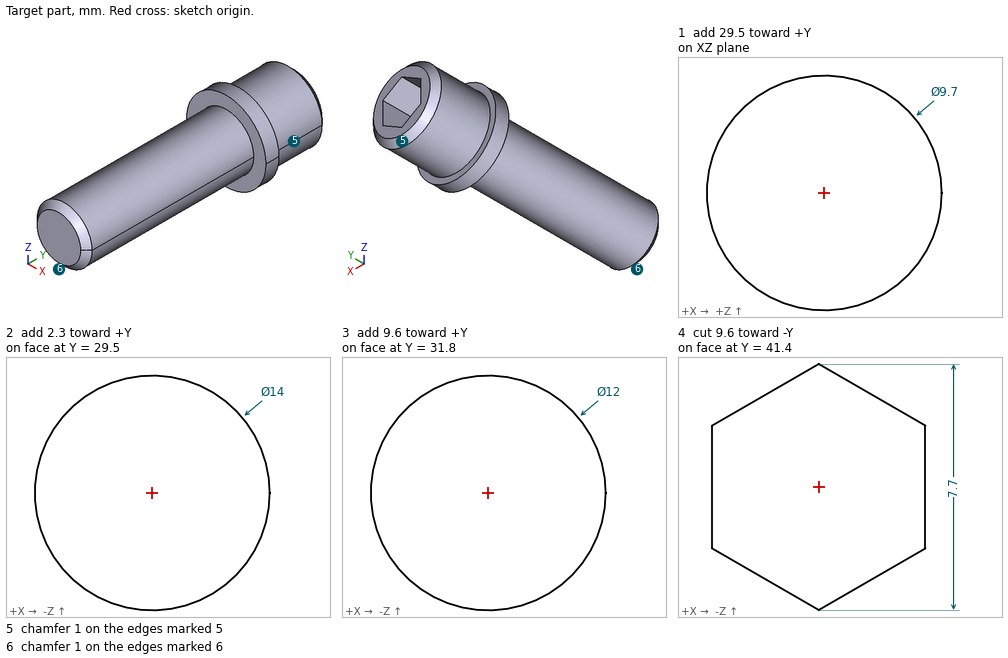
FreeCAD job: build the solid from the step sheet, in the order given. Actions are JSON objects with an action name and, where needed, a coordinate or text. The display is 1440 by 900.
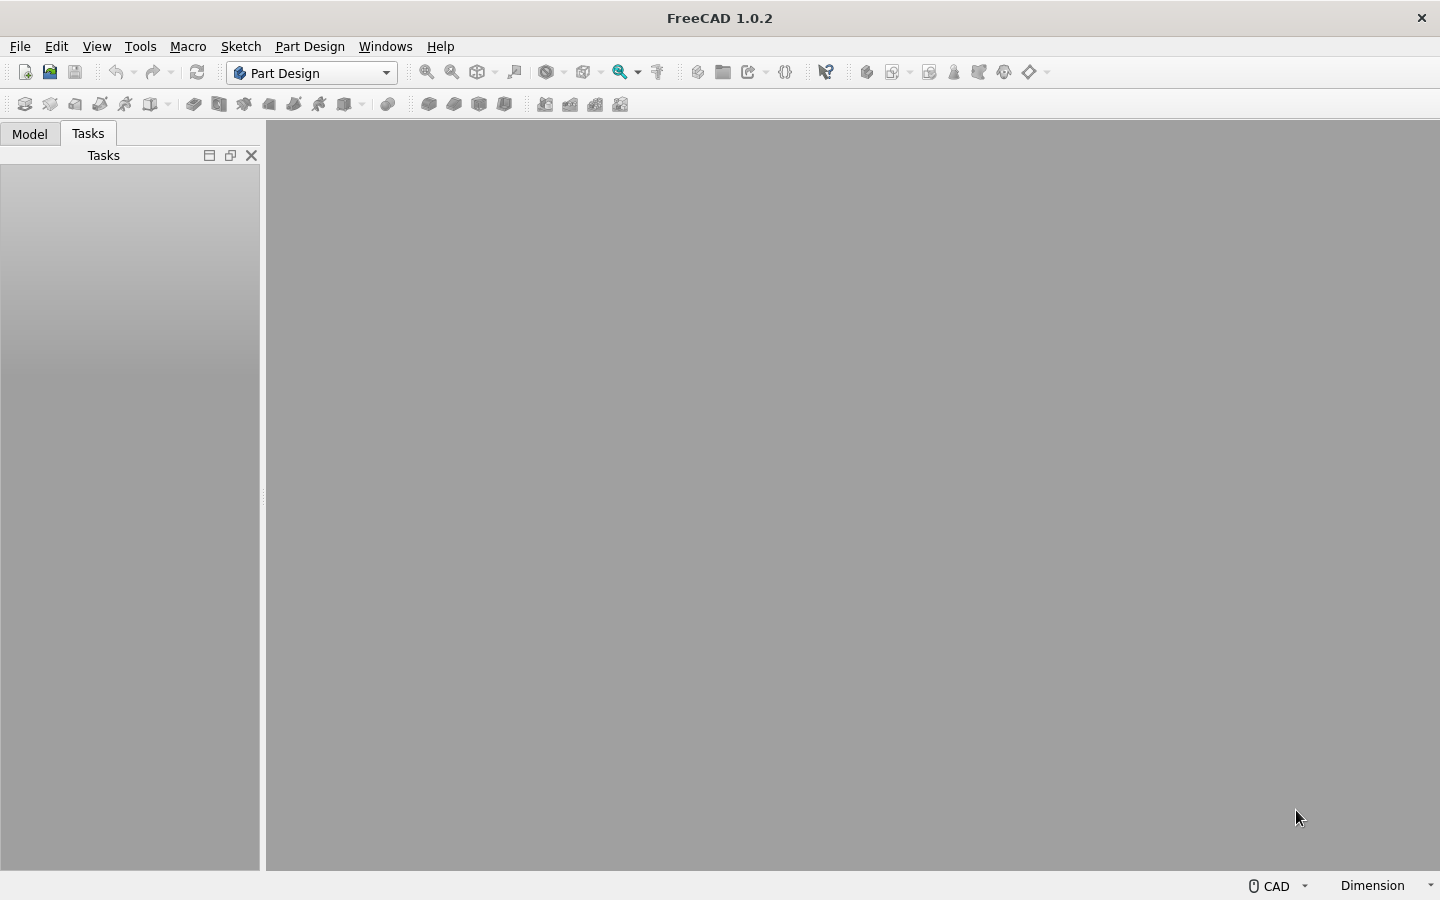
{"action": "left_click", "coordinate": [25, 72]}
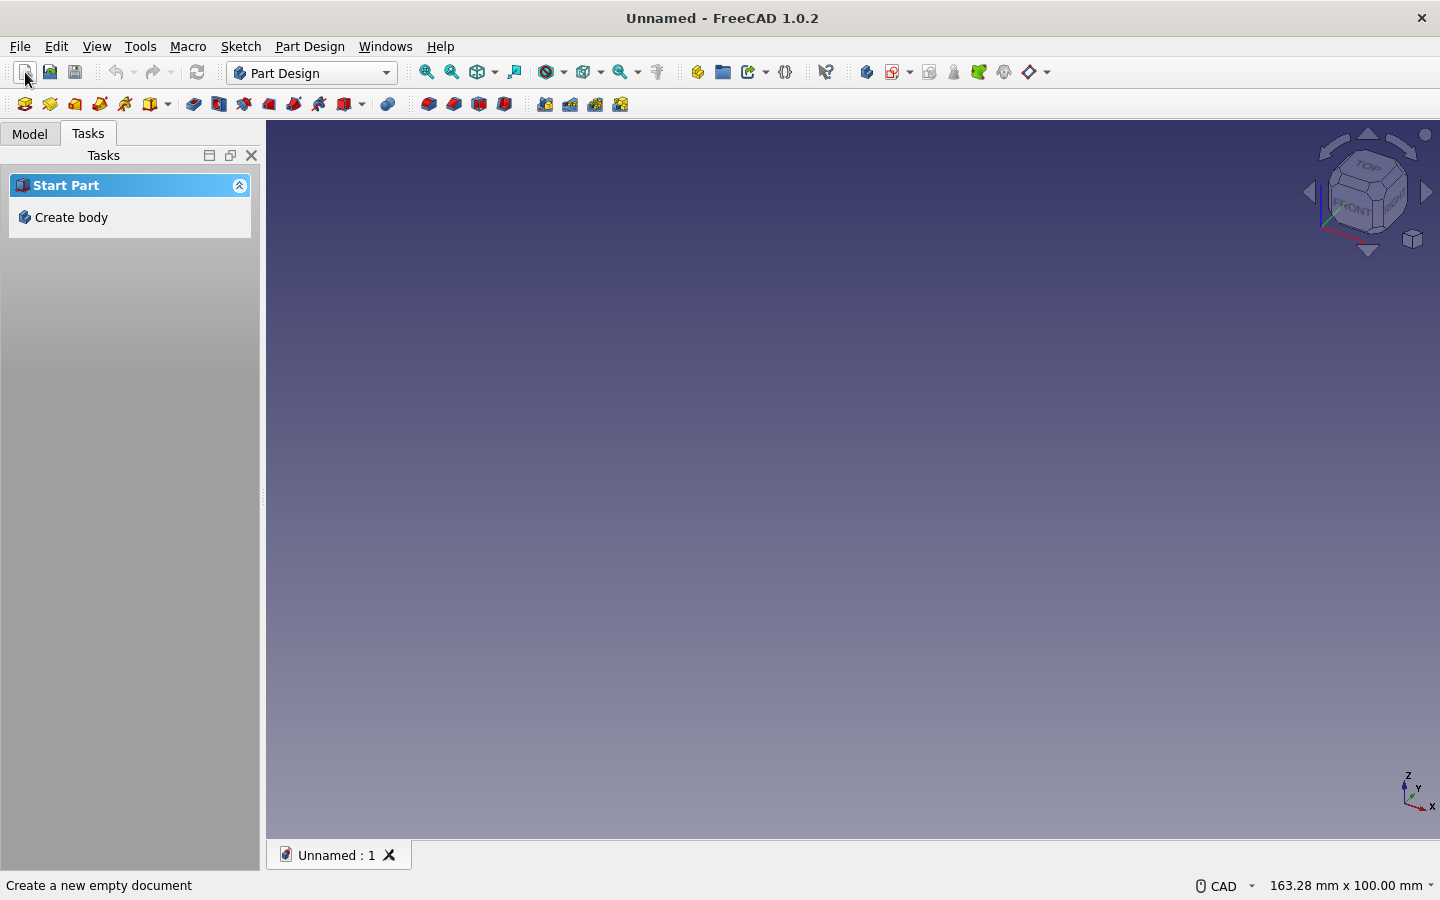
{"action": "left_click", "coordinate": [892, 72]}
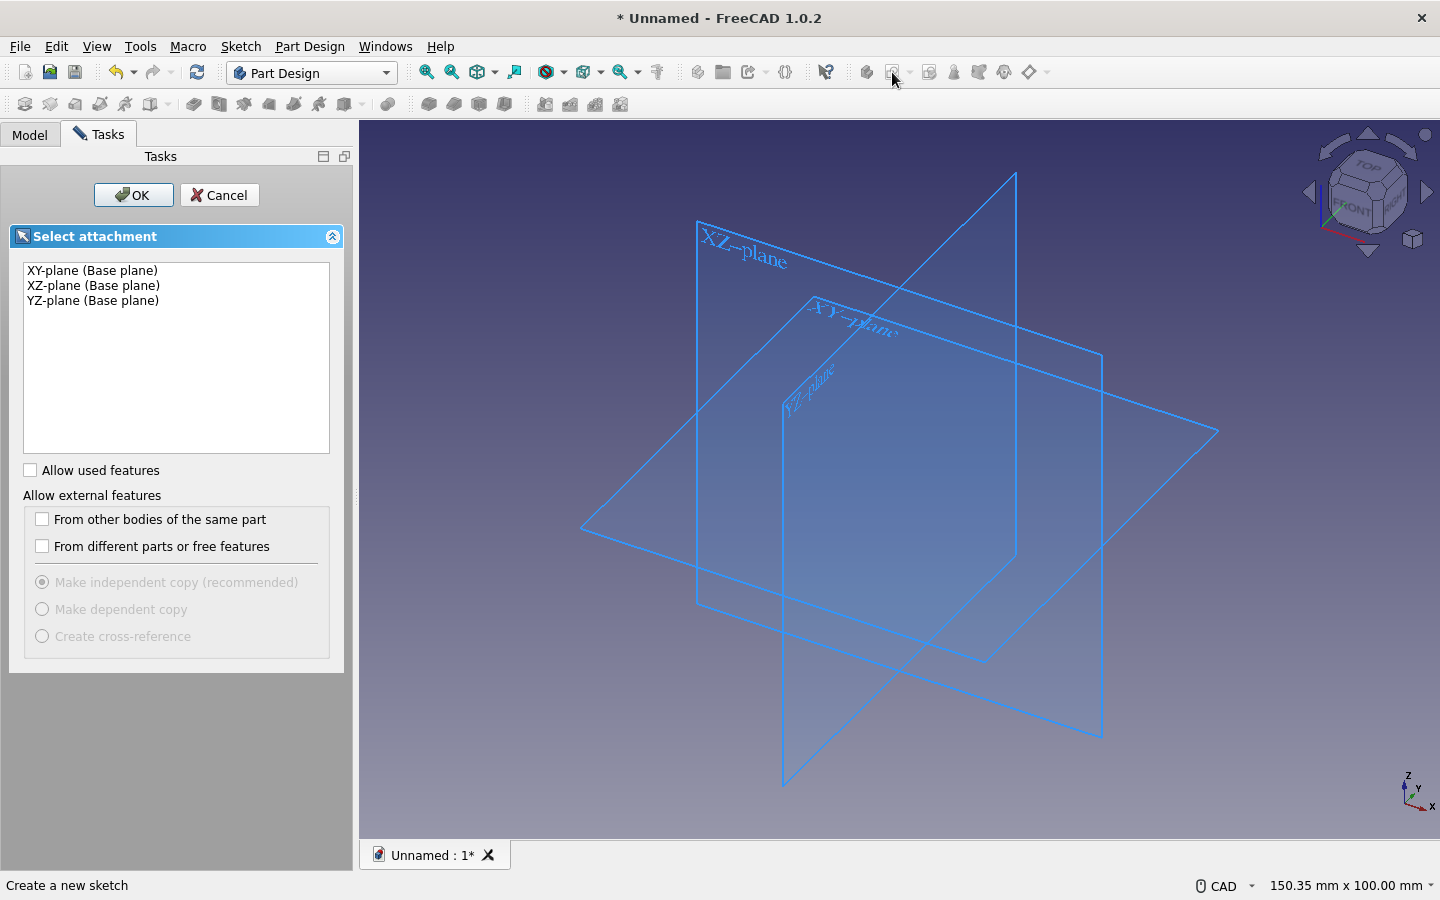
{"action": "left_click", "coordinate": [84, 286]}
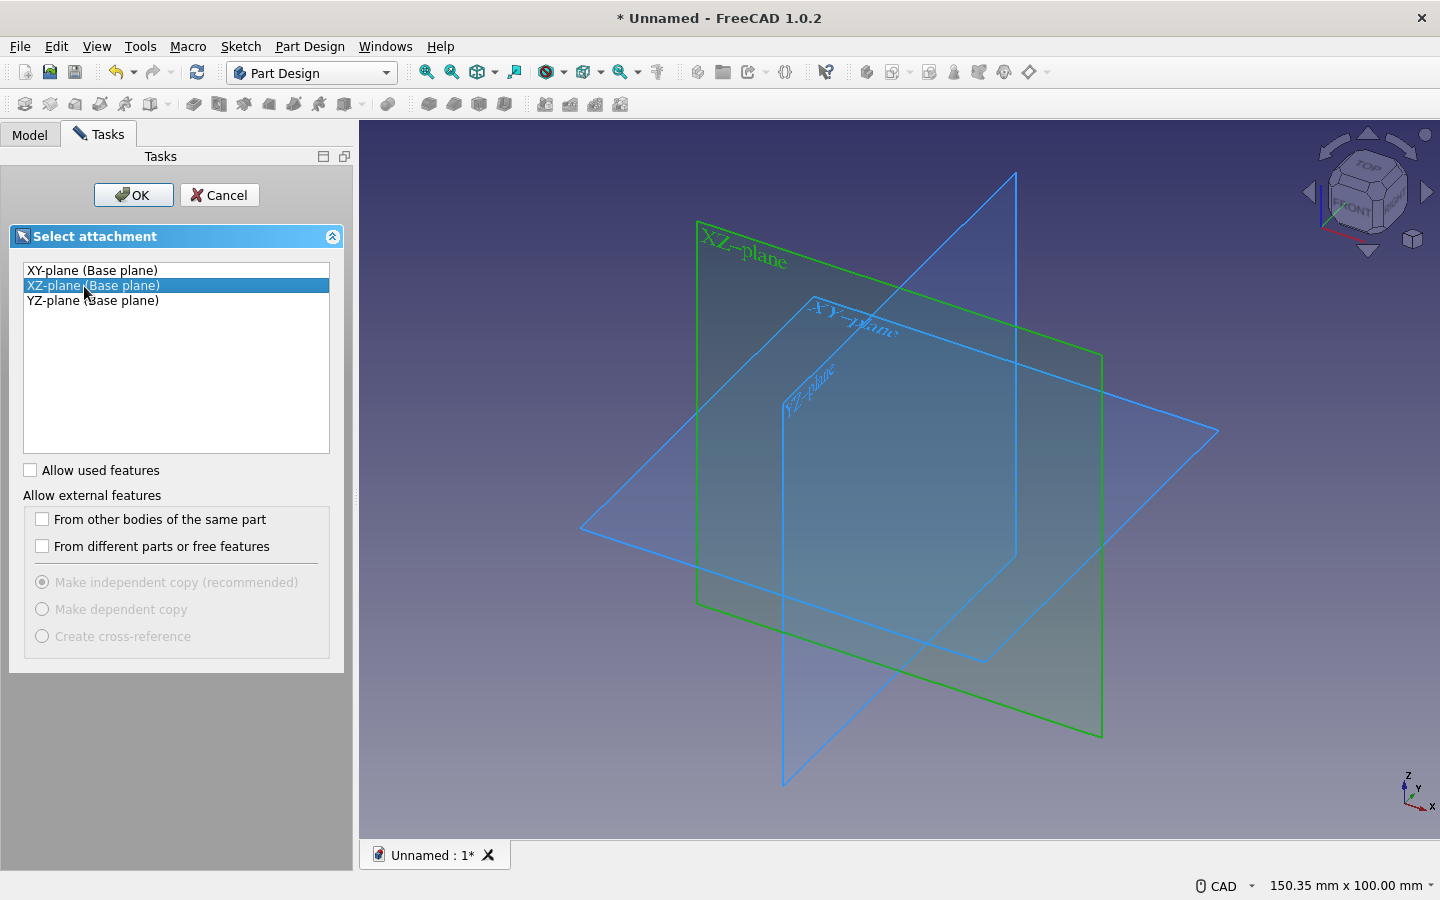
{"action": "left_click", "coordinate": [134, 195]}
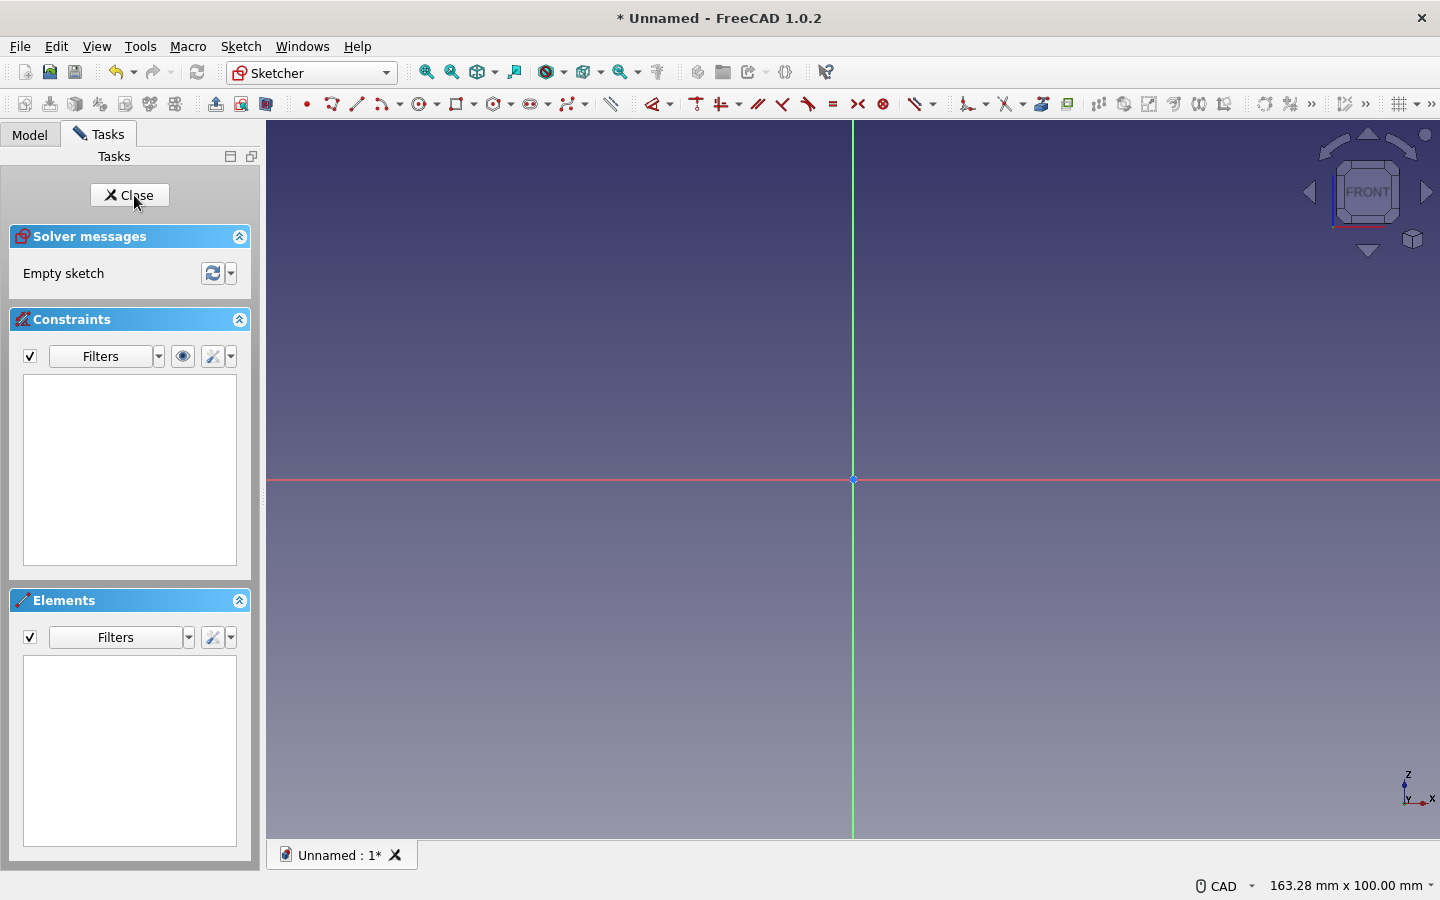
{"action": "scroll", "coordinate": [864, 480], "scroll_direction": "up", "scroll_amount": 10}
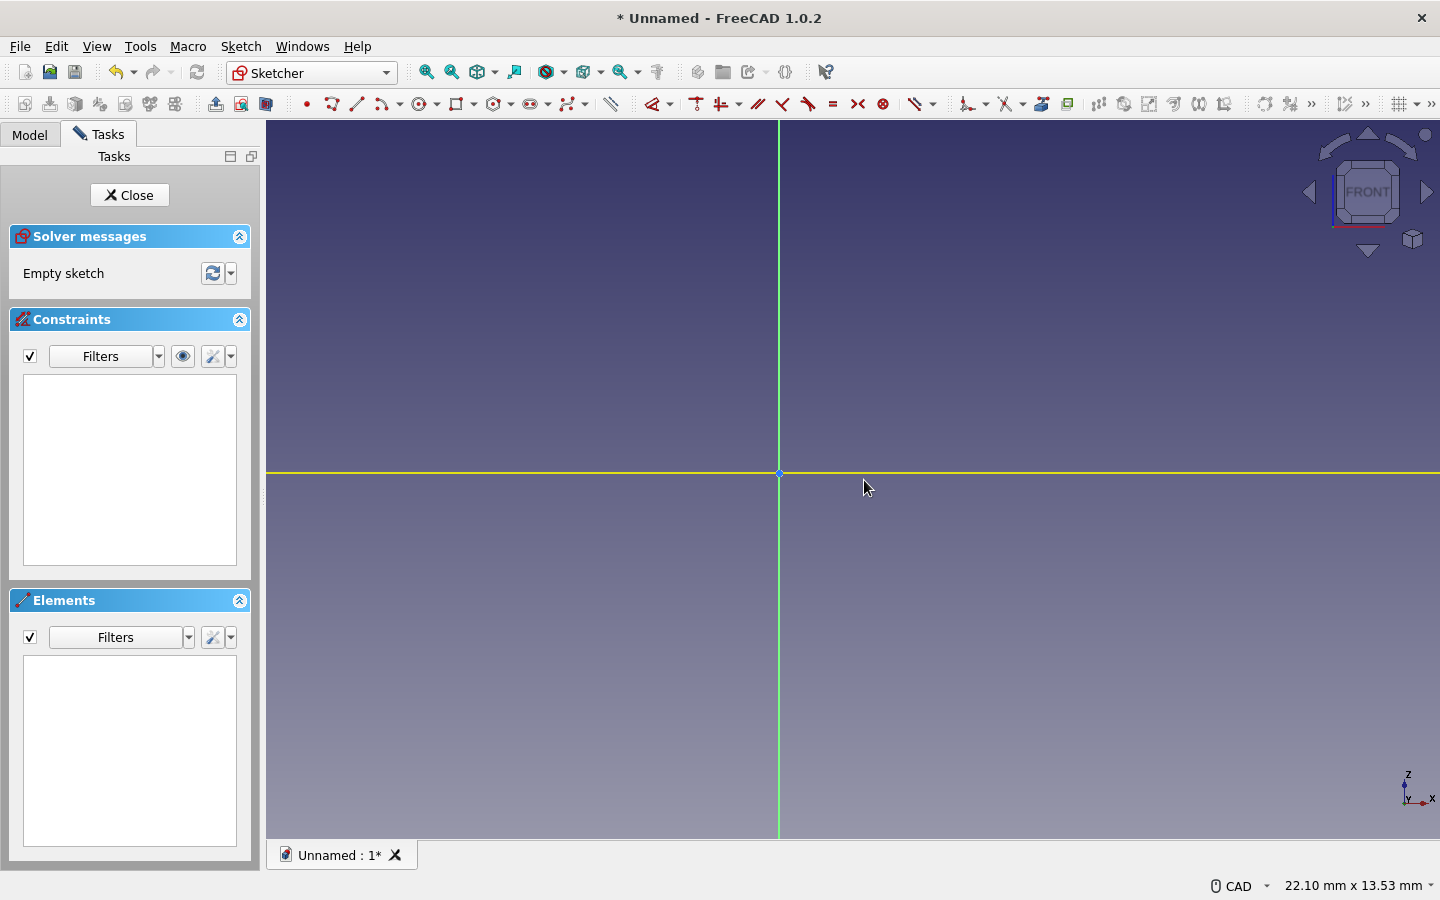
{"action": "left_click", "coordinate": [418, 104]}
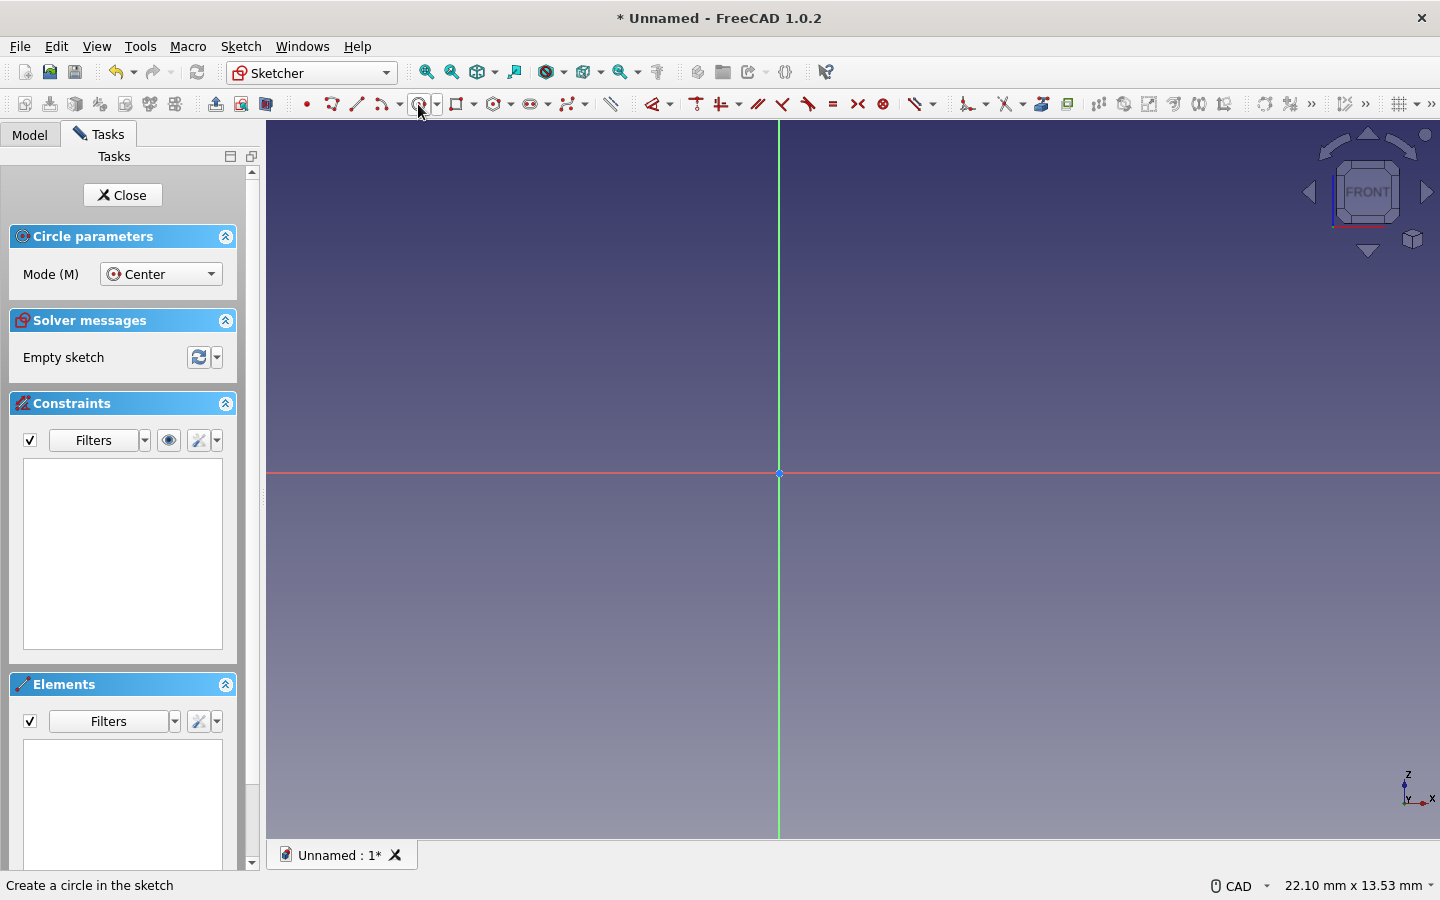
{"action": "left_click", "coordinate": [779, 473]}
{"action": "mouse_move", "coordinate": [962, 291]}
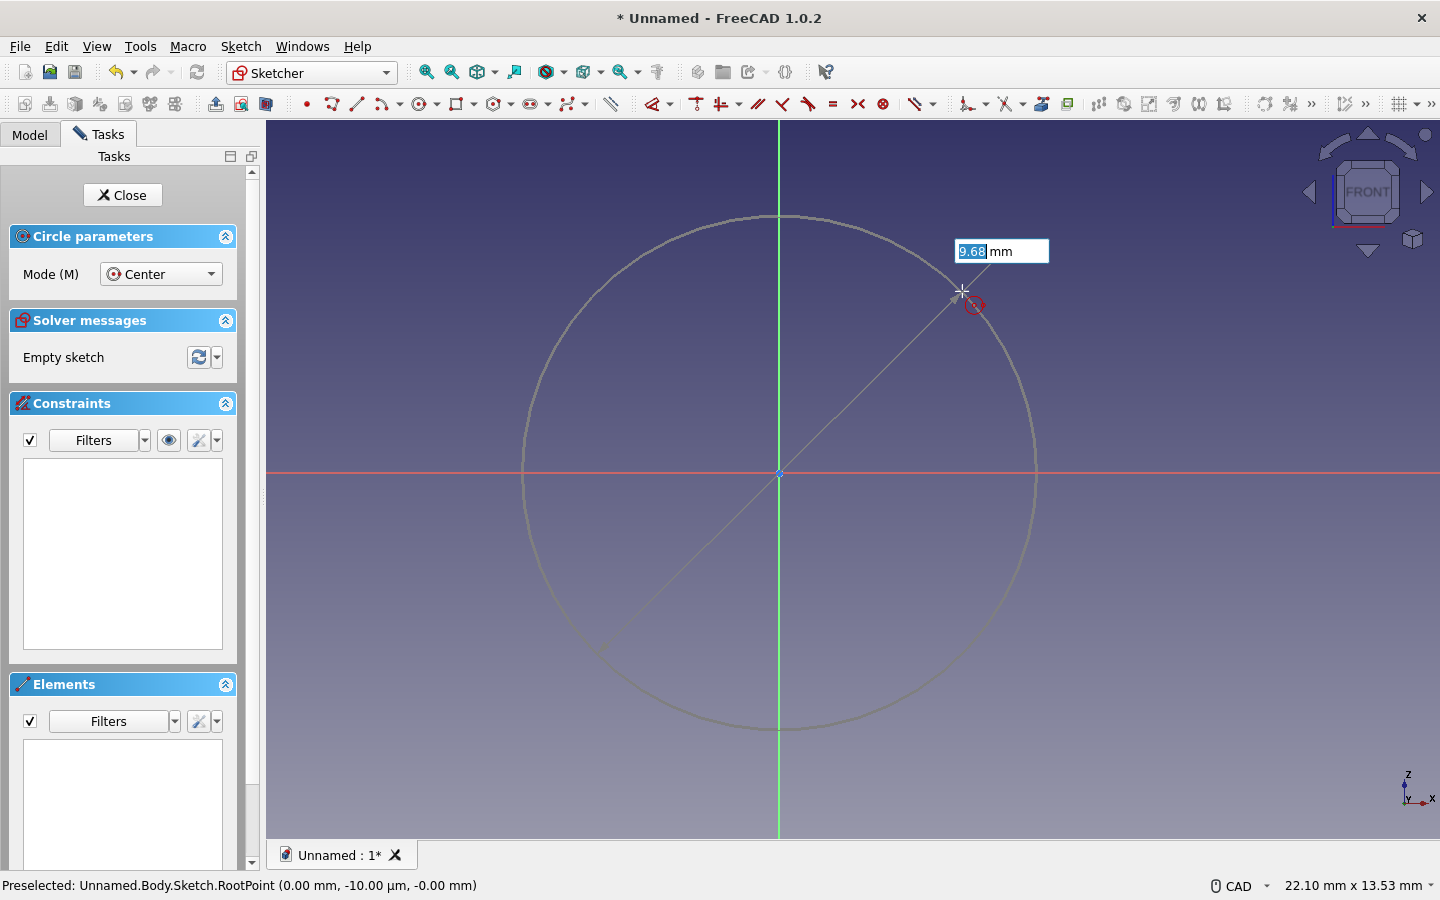
{"action": "type", "text": "9.7"}
{"action": "key", "text": "Return"}
{"action": "key", "text": "Escape"}